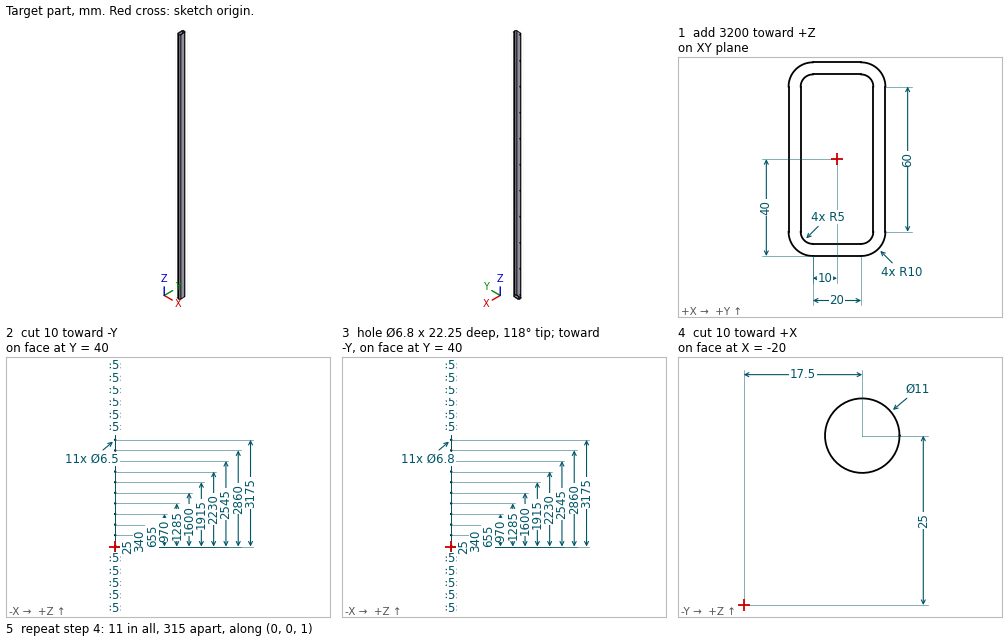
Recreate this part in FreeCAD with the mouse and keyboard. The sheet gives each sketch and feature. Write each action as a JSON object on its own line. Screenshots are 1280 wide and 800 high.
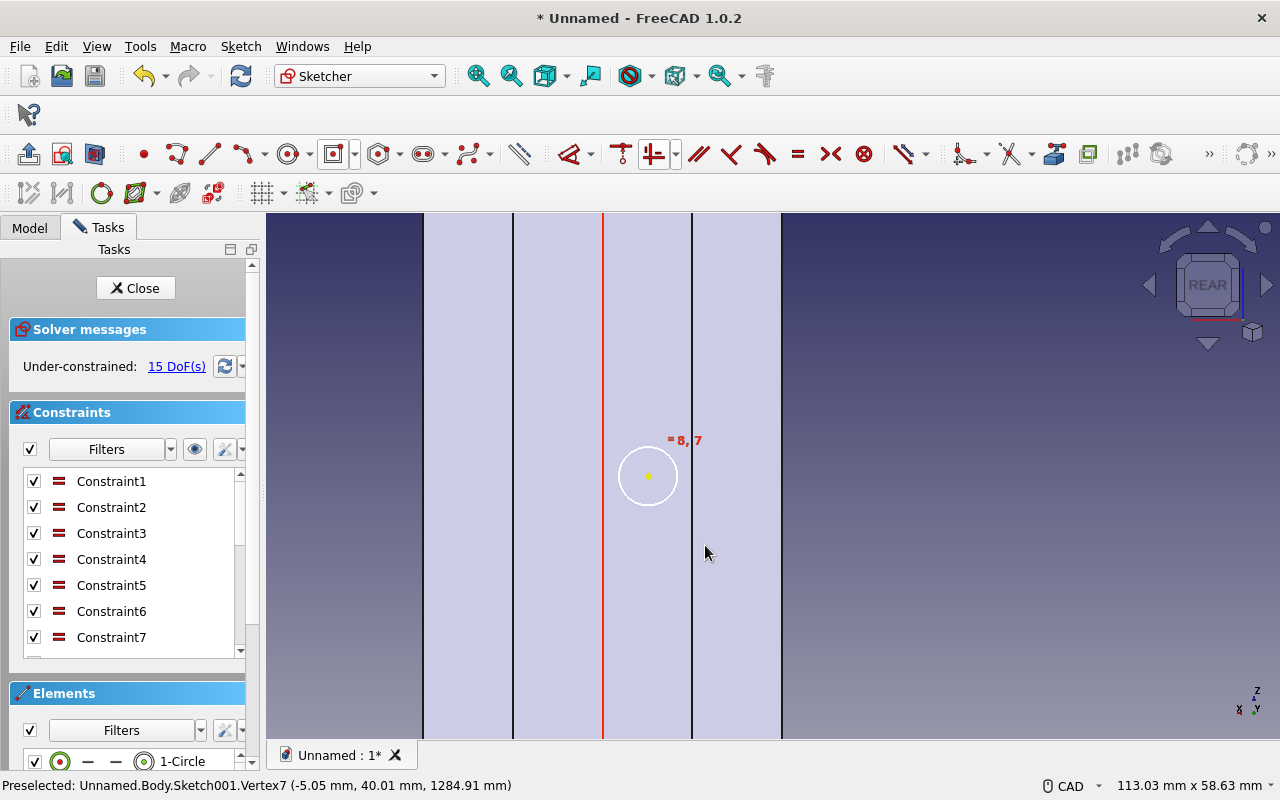
{"action": "left_click", "coordinate": [648, 476]}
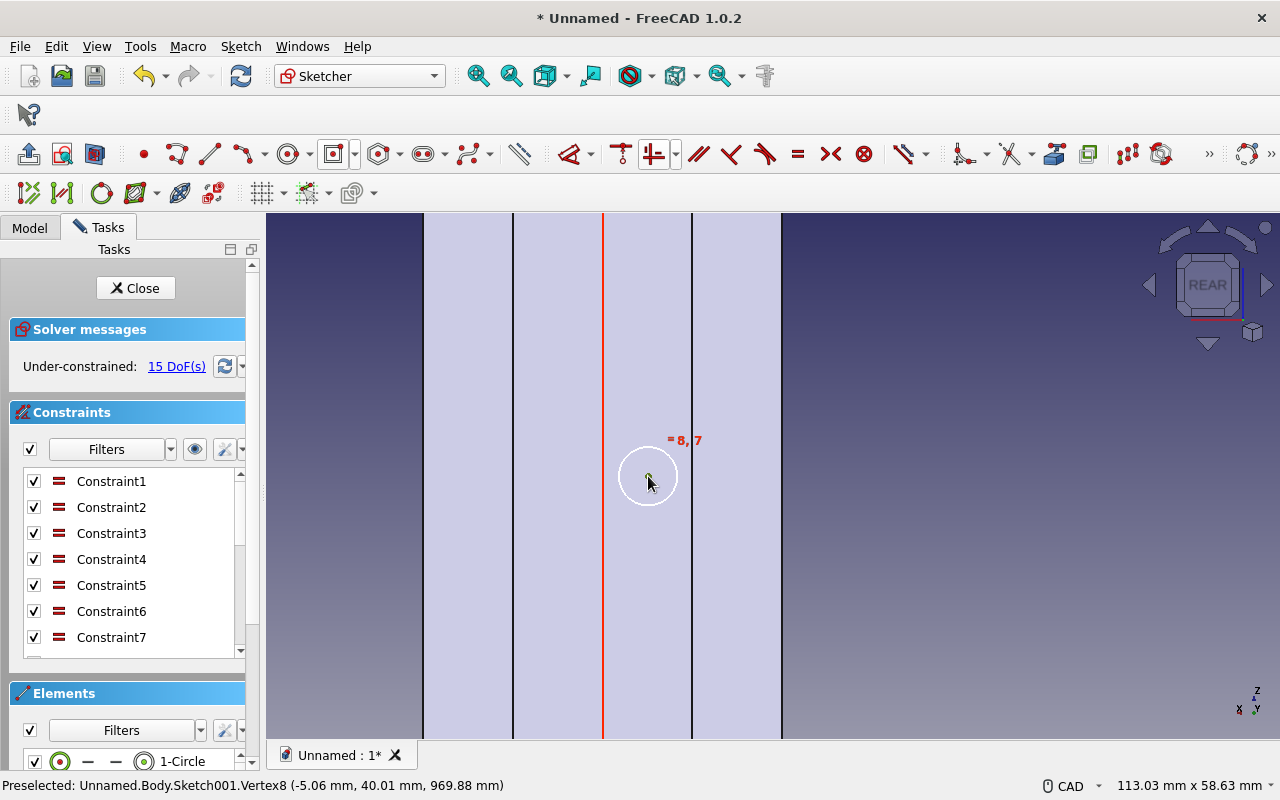
{"action": "key", "text": "l"}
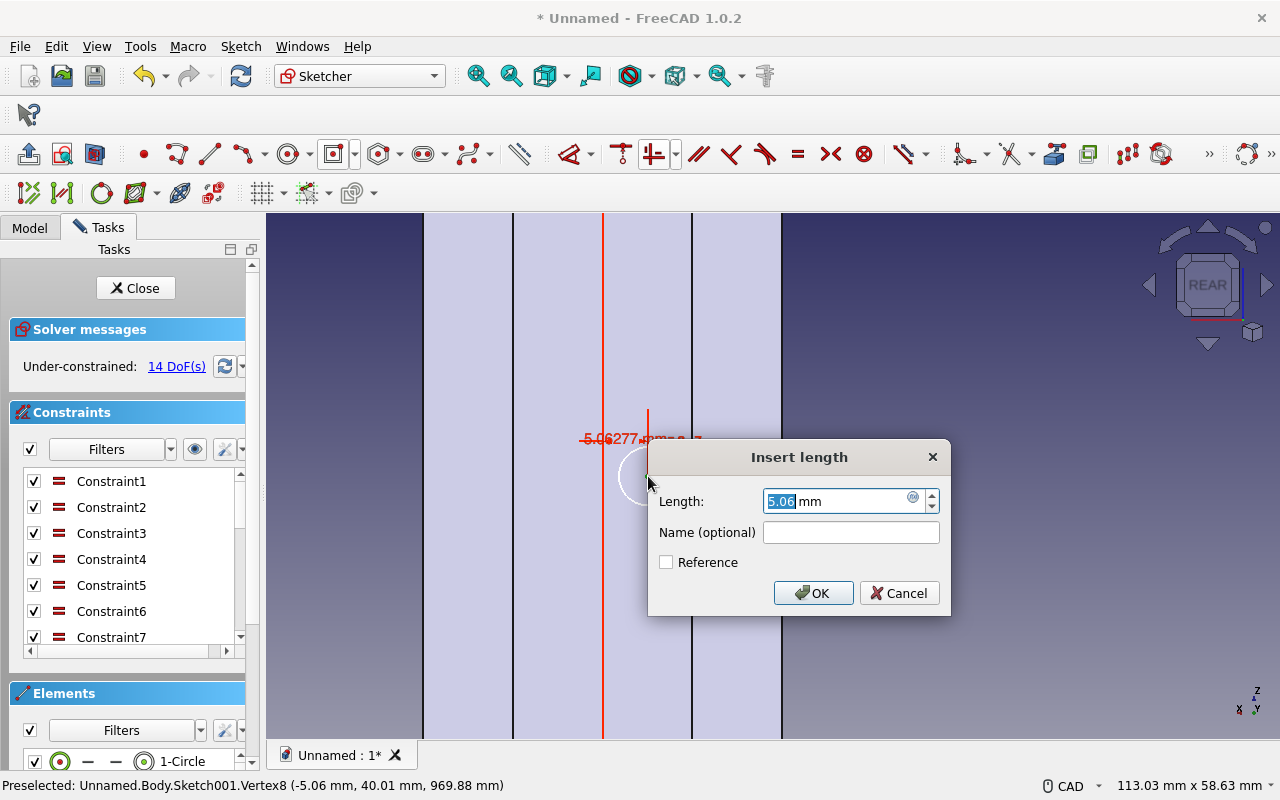
{"action": "type", "text": "5"}
{"action": "key", "text": "Return"}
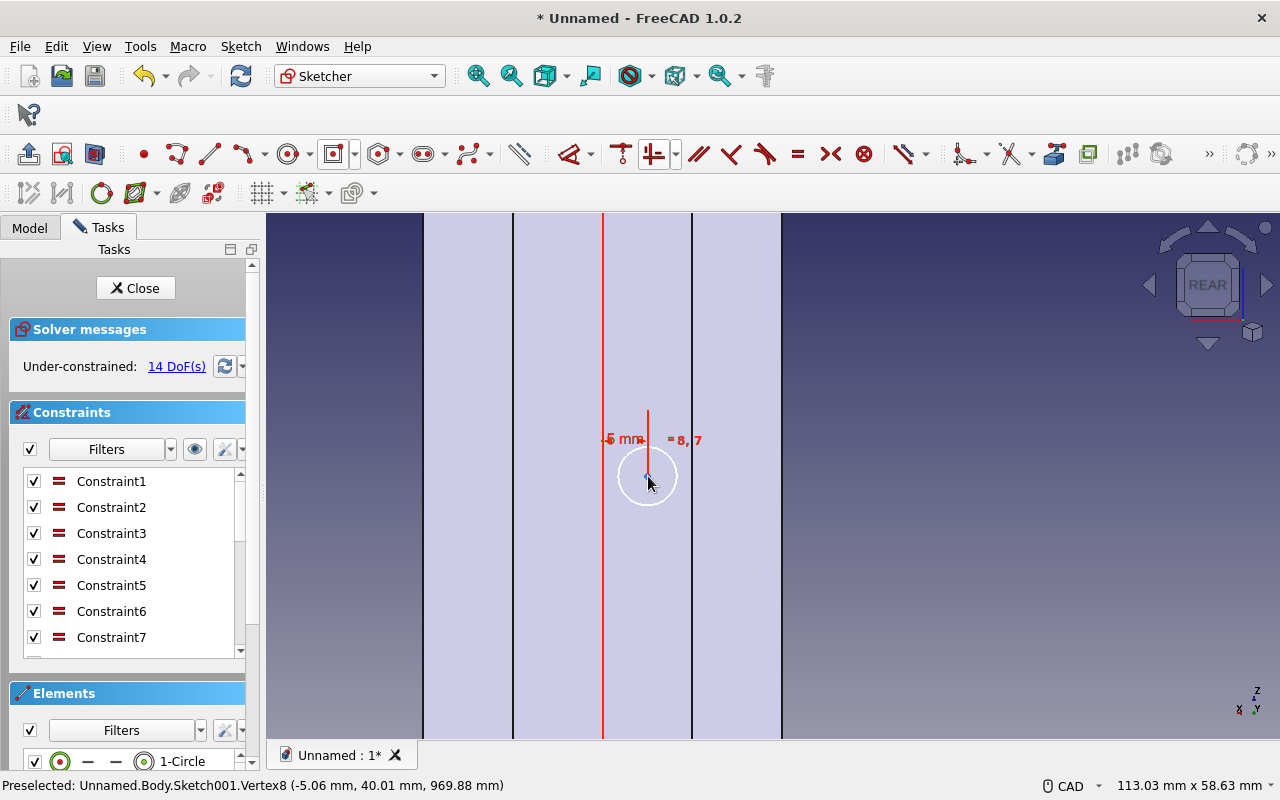
{"action": "scroll", "coordinate": [704, 476], "scroll_direction": "down", "scroll_amount": 15}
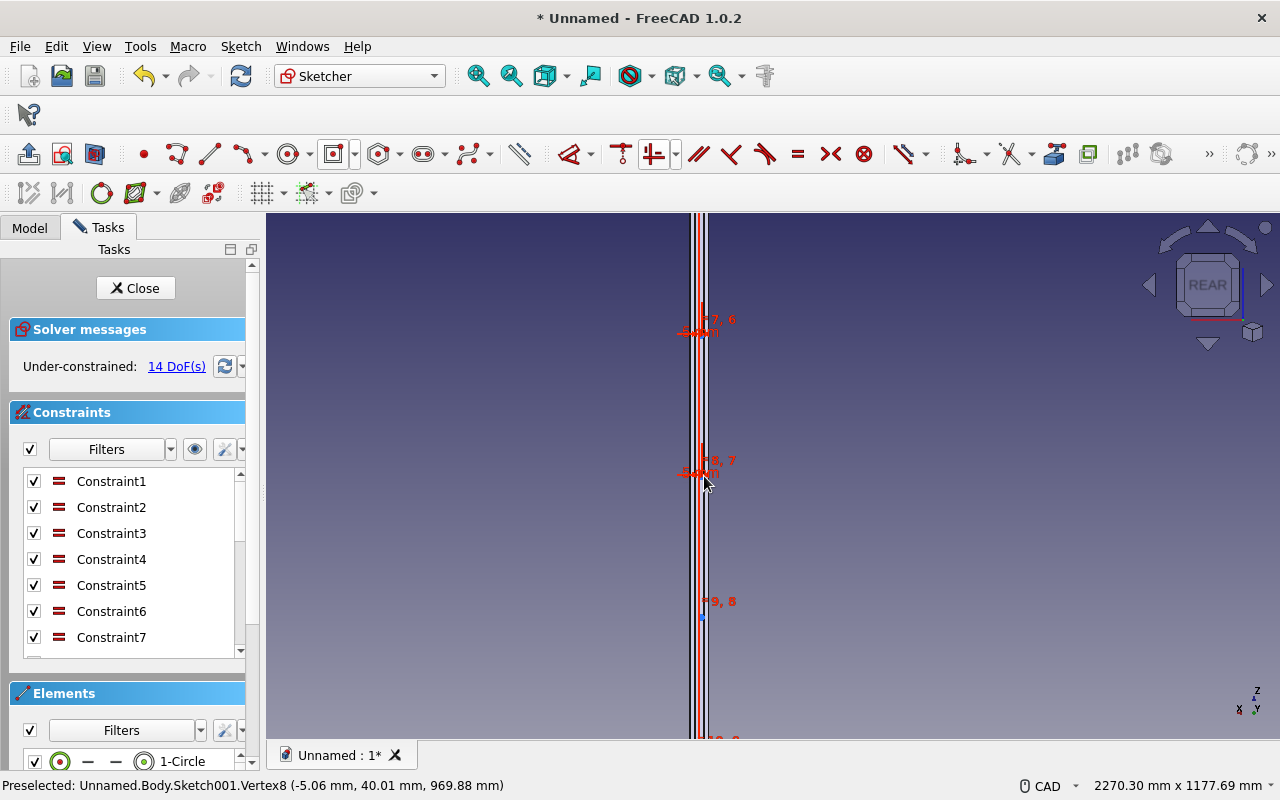
{"action": "scroll", "coordinate": [706, 566], "scroll_direction": "down", "scroll_amount": 7}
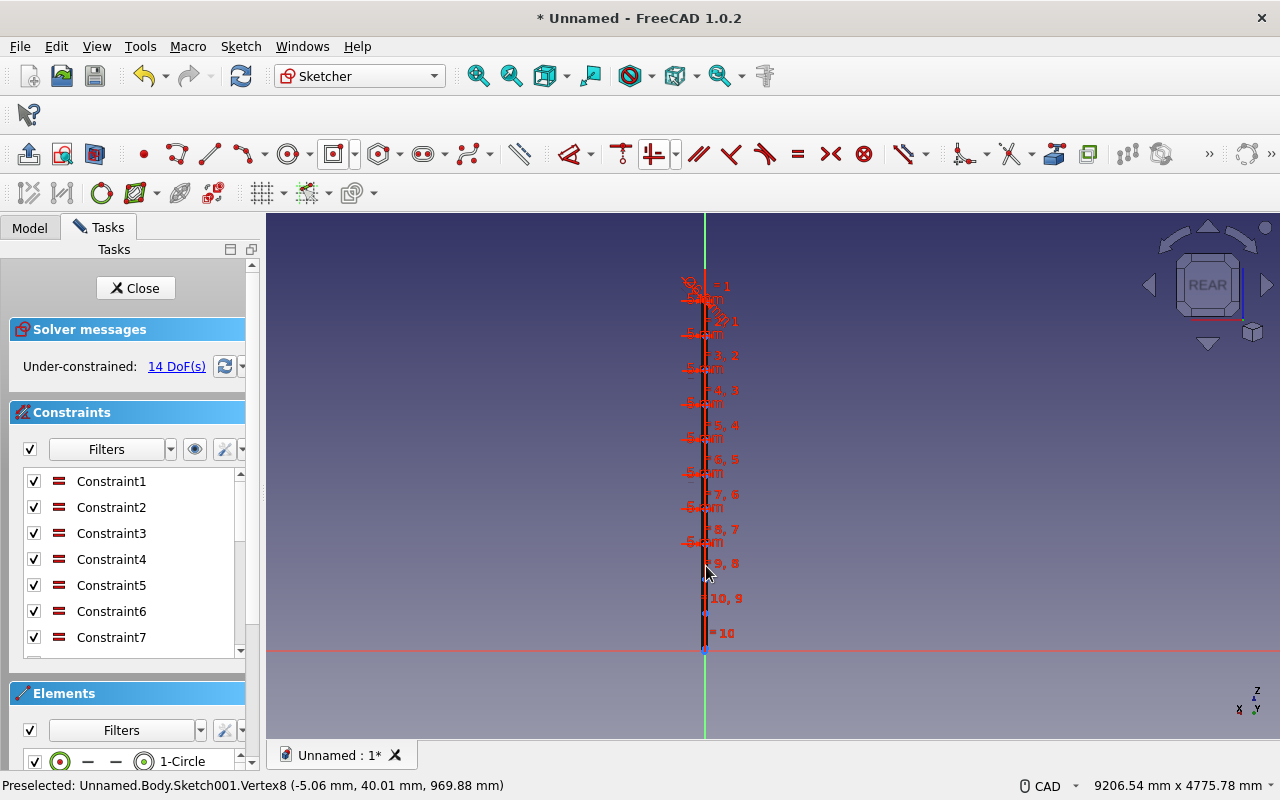
{"action": "scroll", "coordinate": [705, 579], "scroll_direction": "up", "scroll_amount": 22}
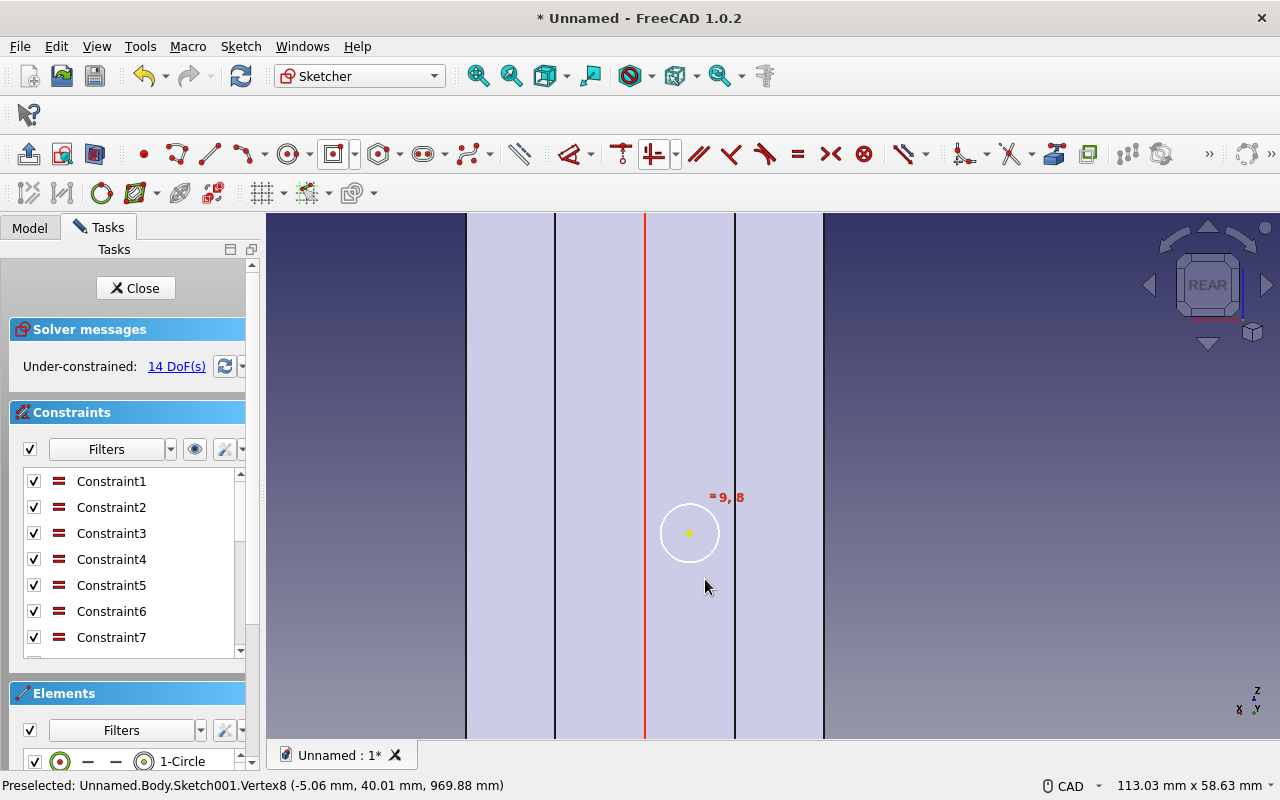
{"action": "left_click", "coordinate": [690, 533]}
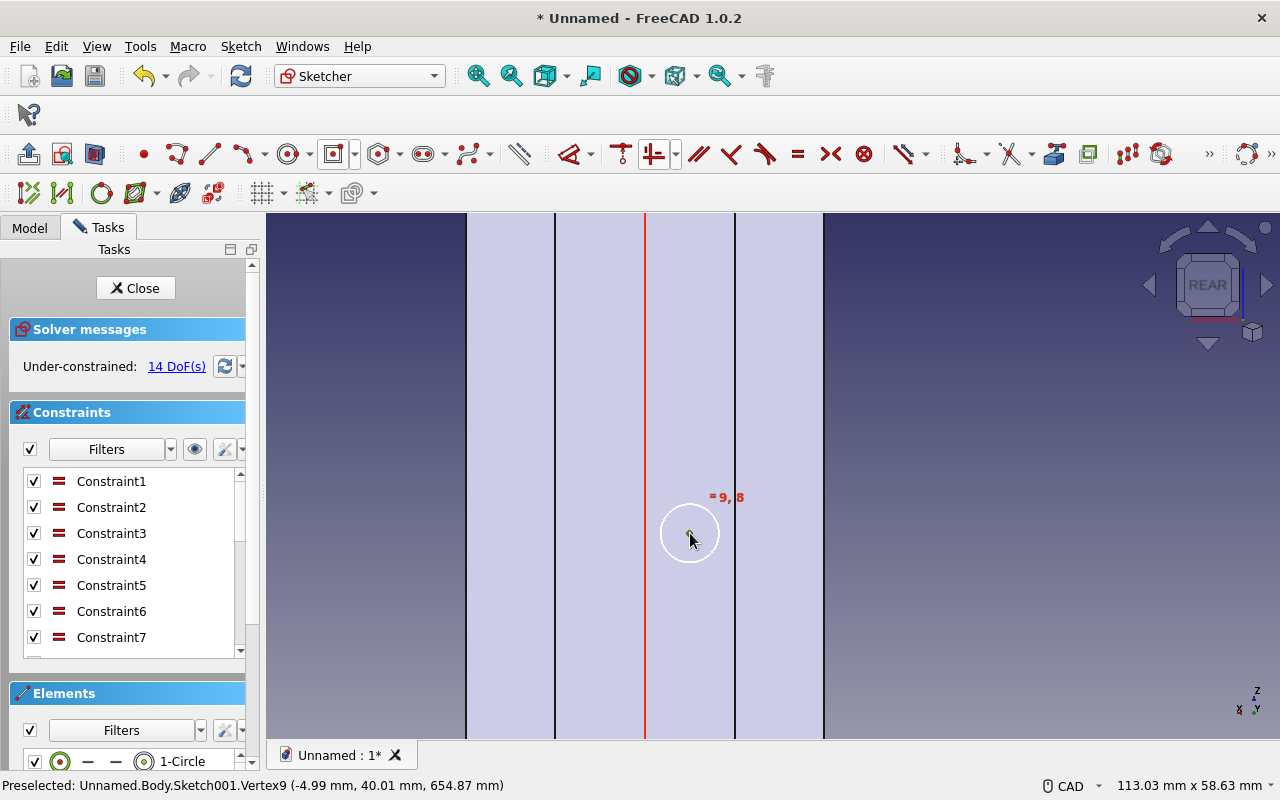
{"action": "left_click", "coordinate": [590, 154]}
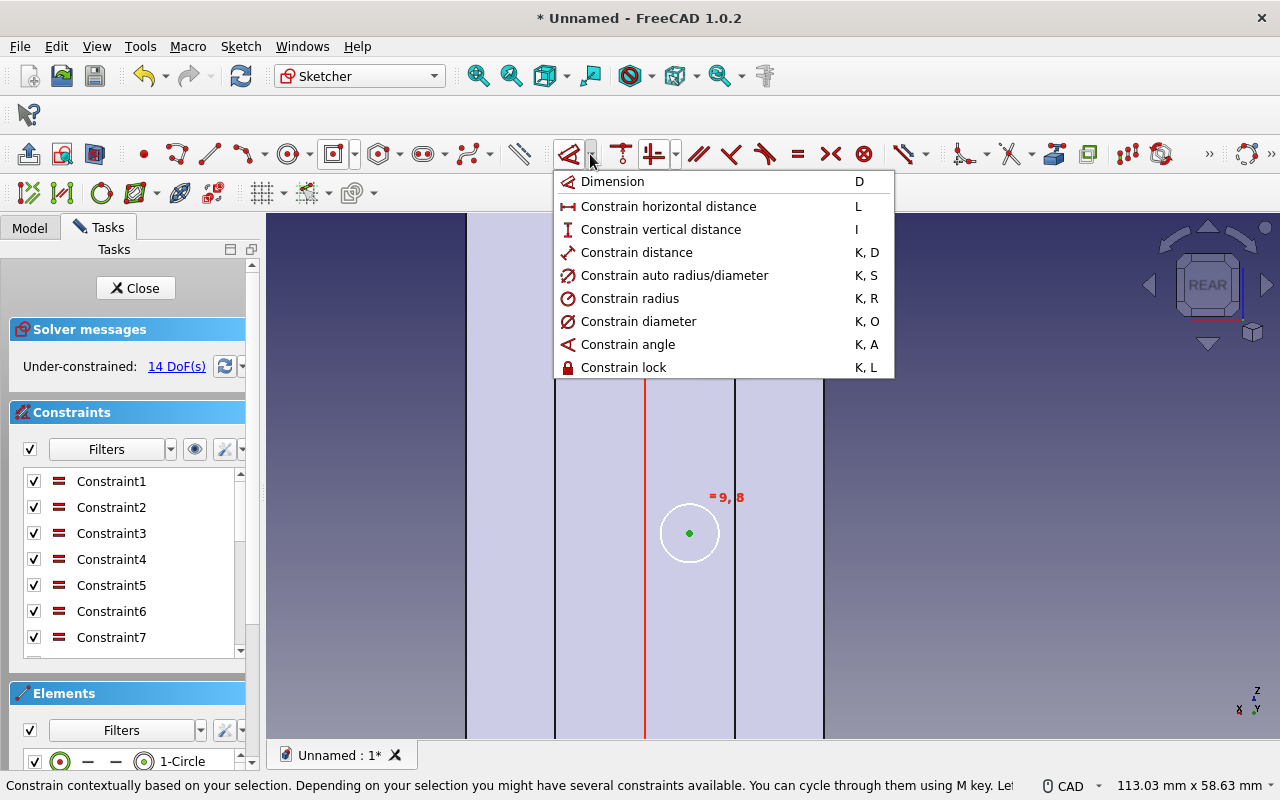
{"action": "left_click", "coordinate": [724, 206]}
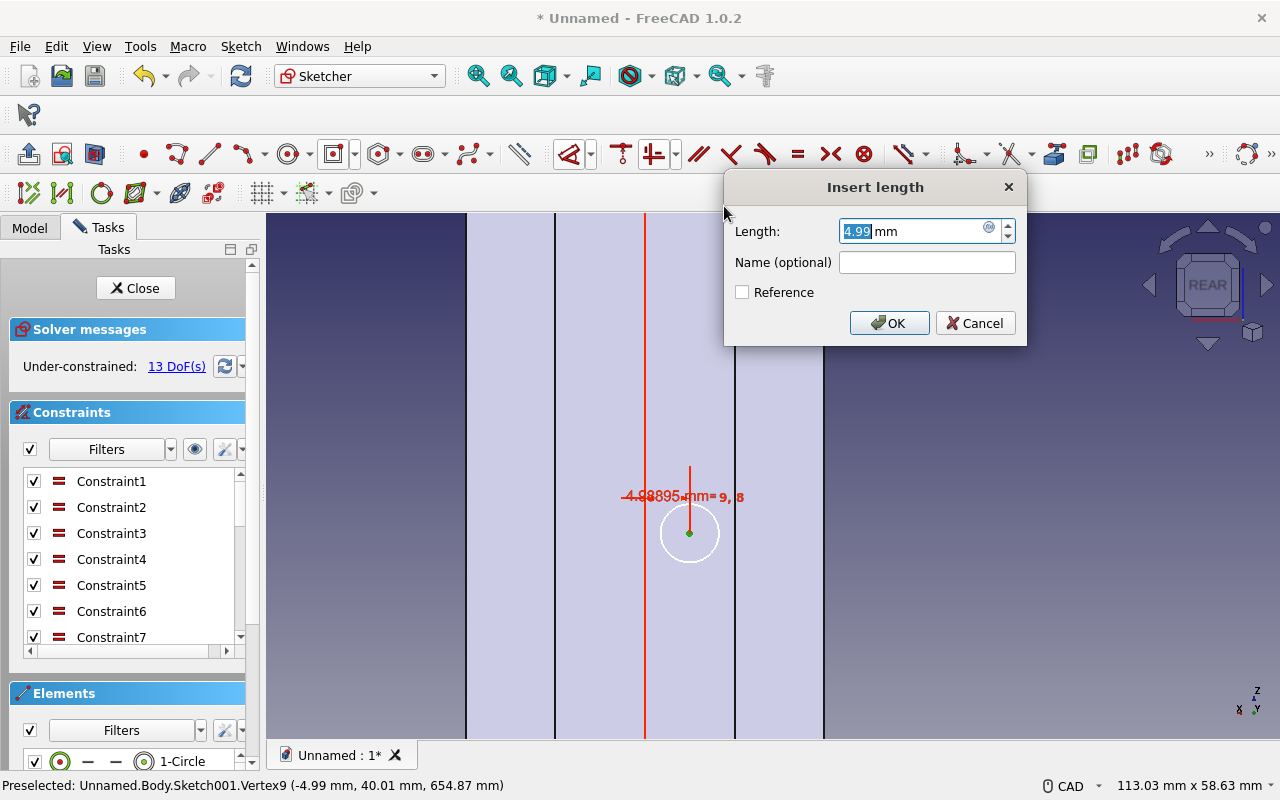
{"action": "type", "text": "5"}
{"action": "key", "text": "Return"}